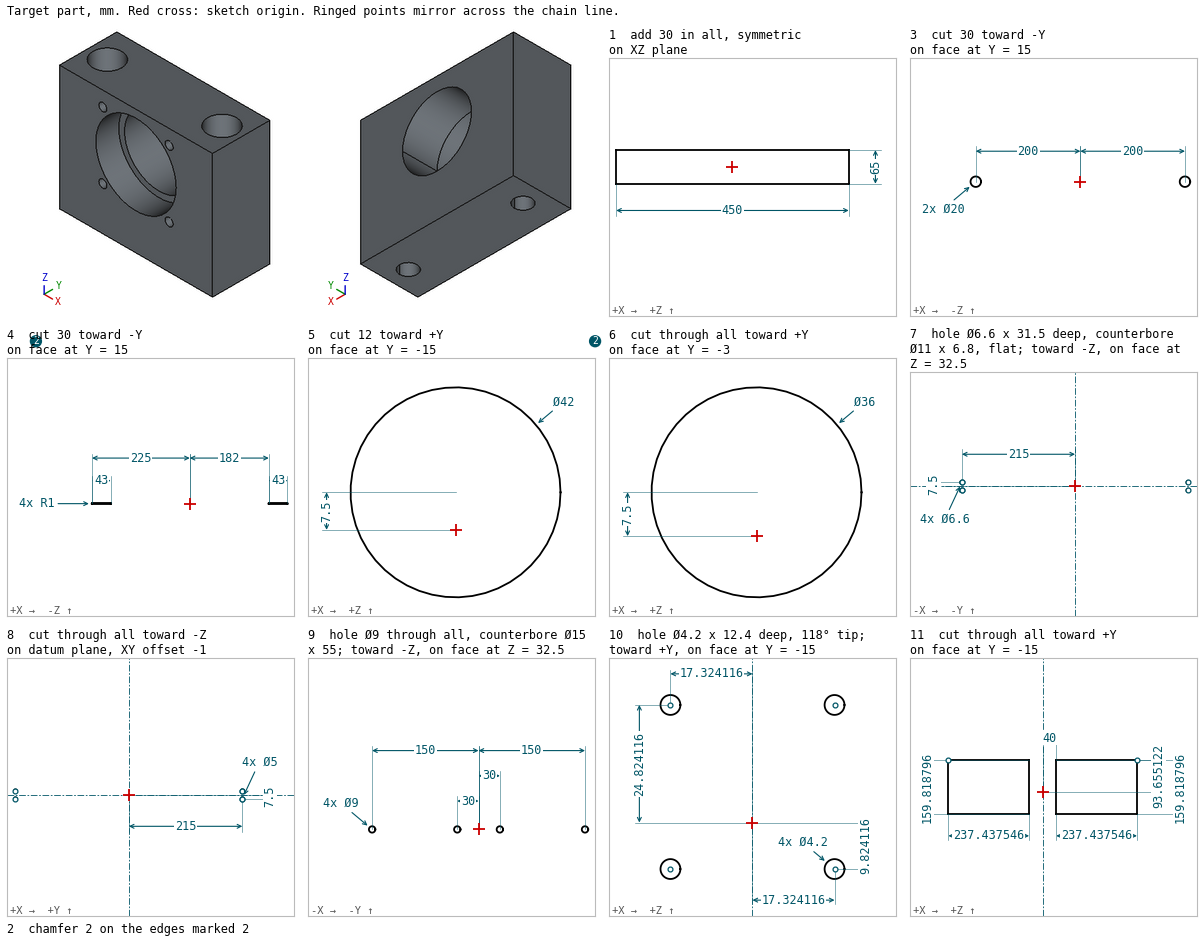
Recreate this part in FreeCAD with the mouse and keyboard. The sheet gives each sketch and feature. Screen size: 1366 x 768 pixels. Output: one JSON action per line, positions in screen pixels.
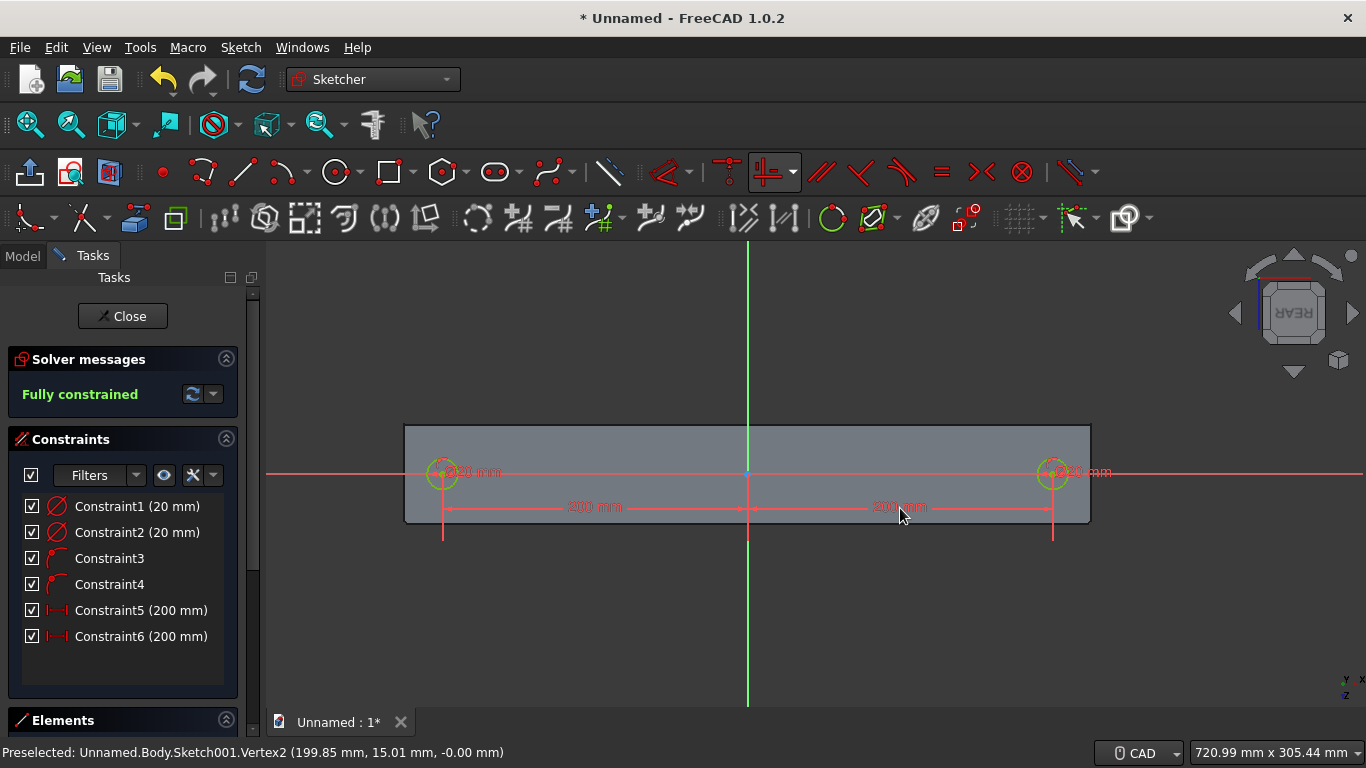
{"action": "left_click", "coordinate": [123, 316]}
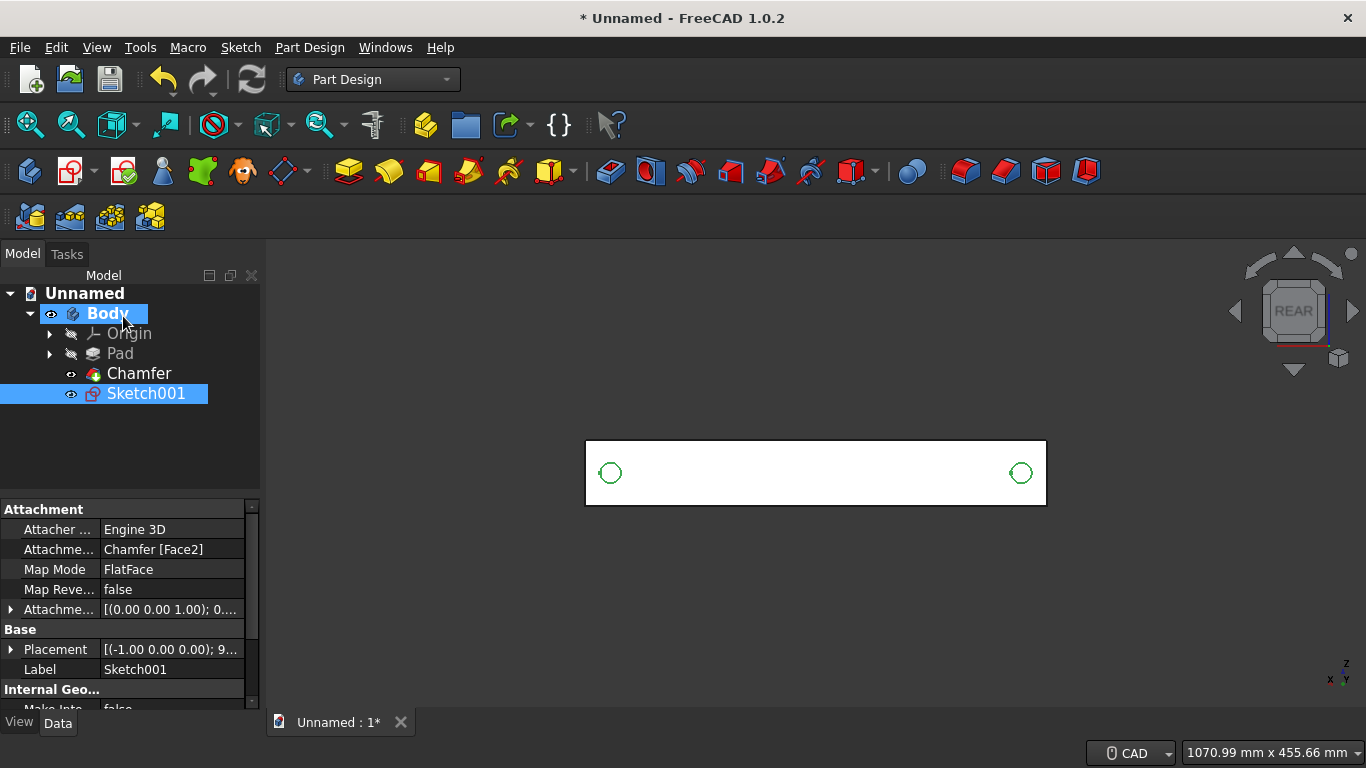
{"action": "left_click", "coordinate": [612, 172]}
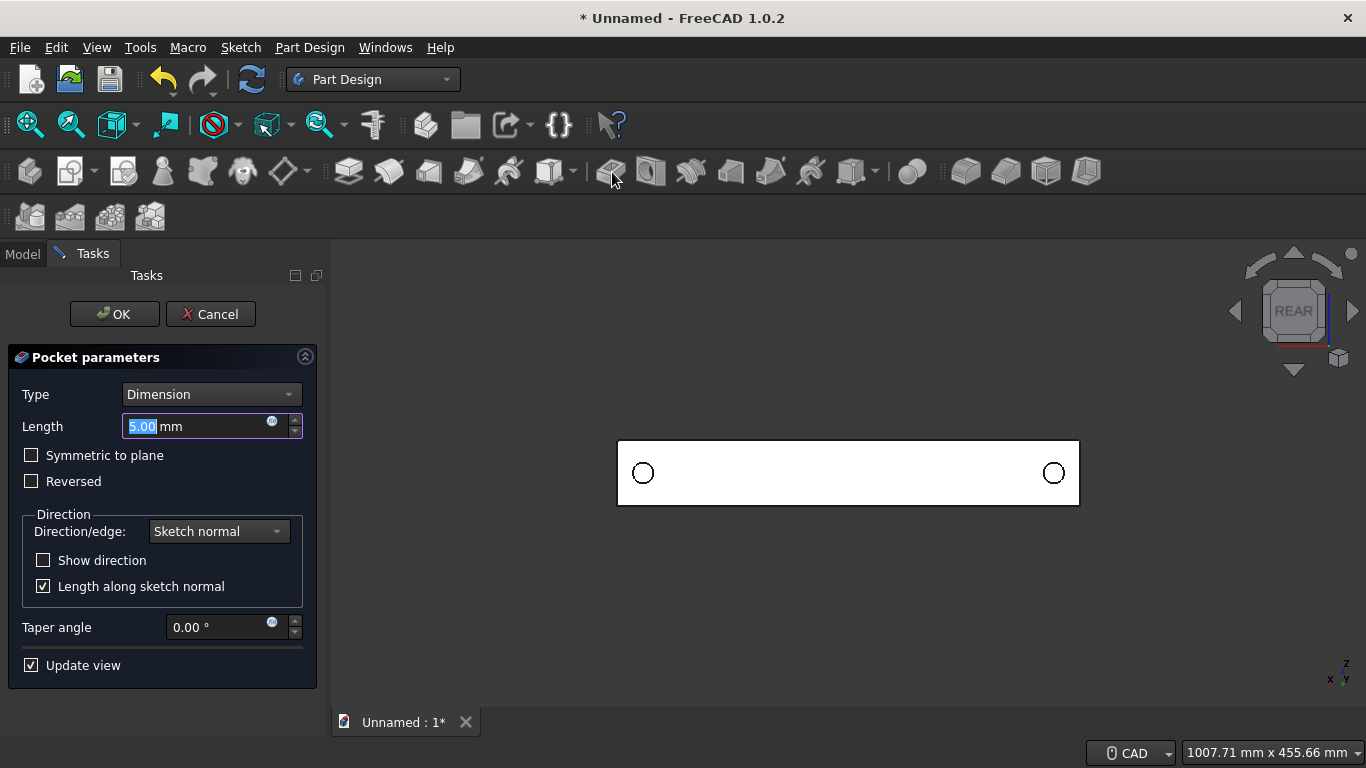
{"action": "type", "text": "30"}
{"action": "key", "text": "Tab"}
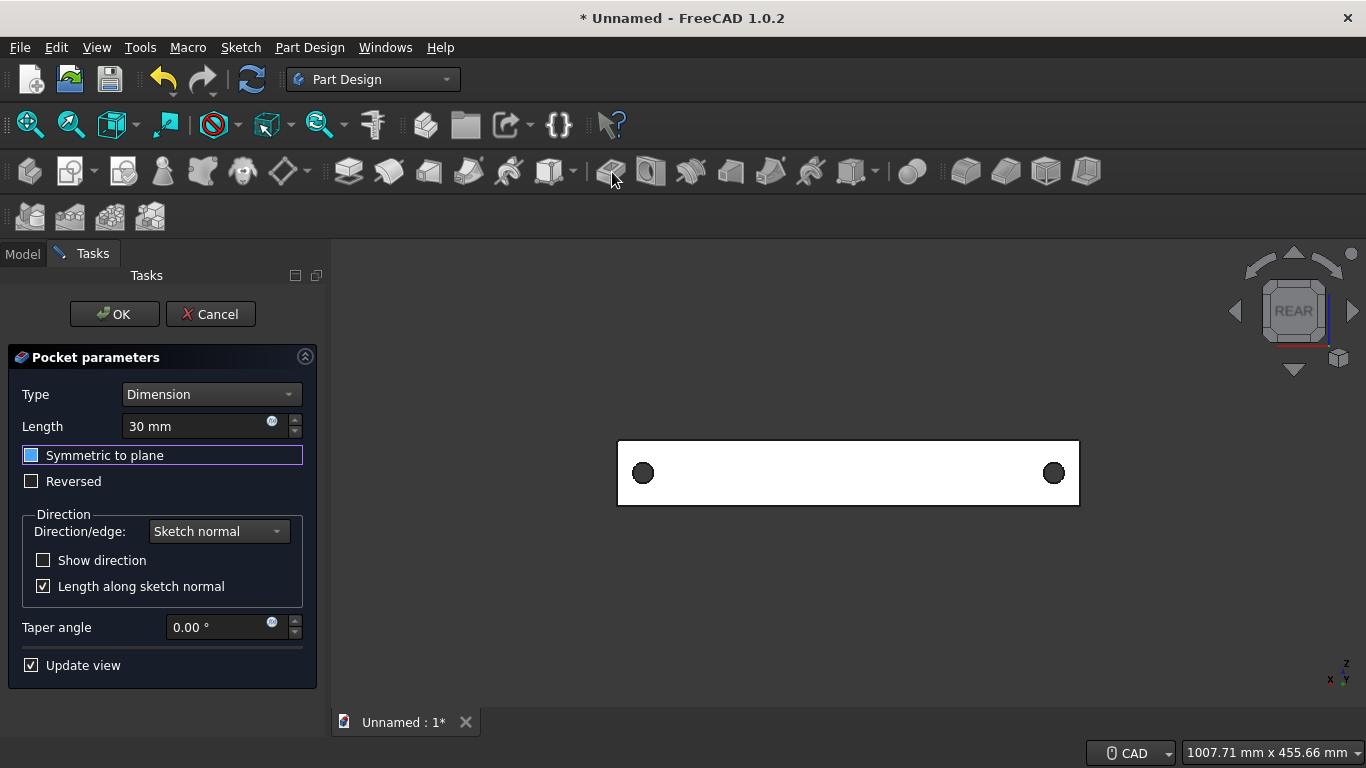
{"action": "left_click", "coordinate": [115, 314]}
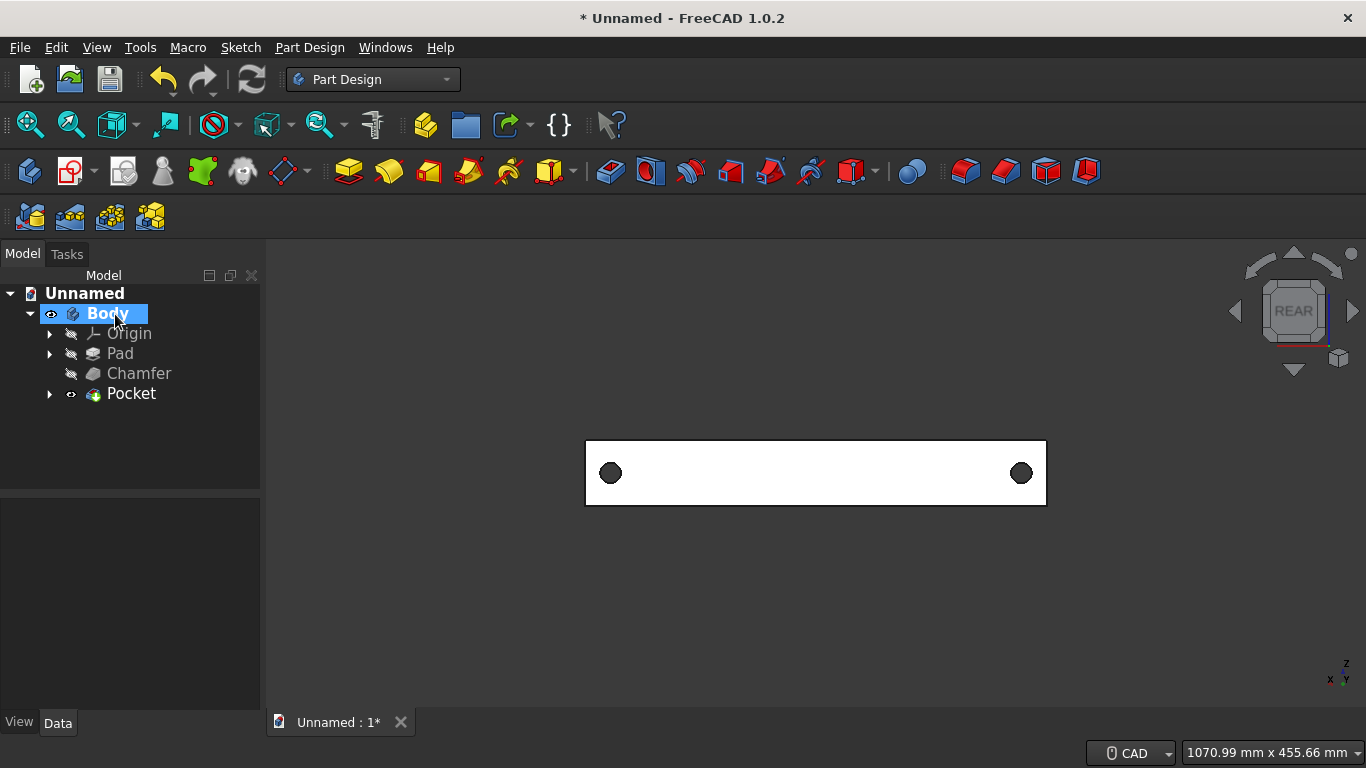
{"action": "key", "text": "v f"}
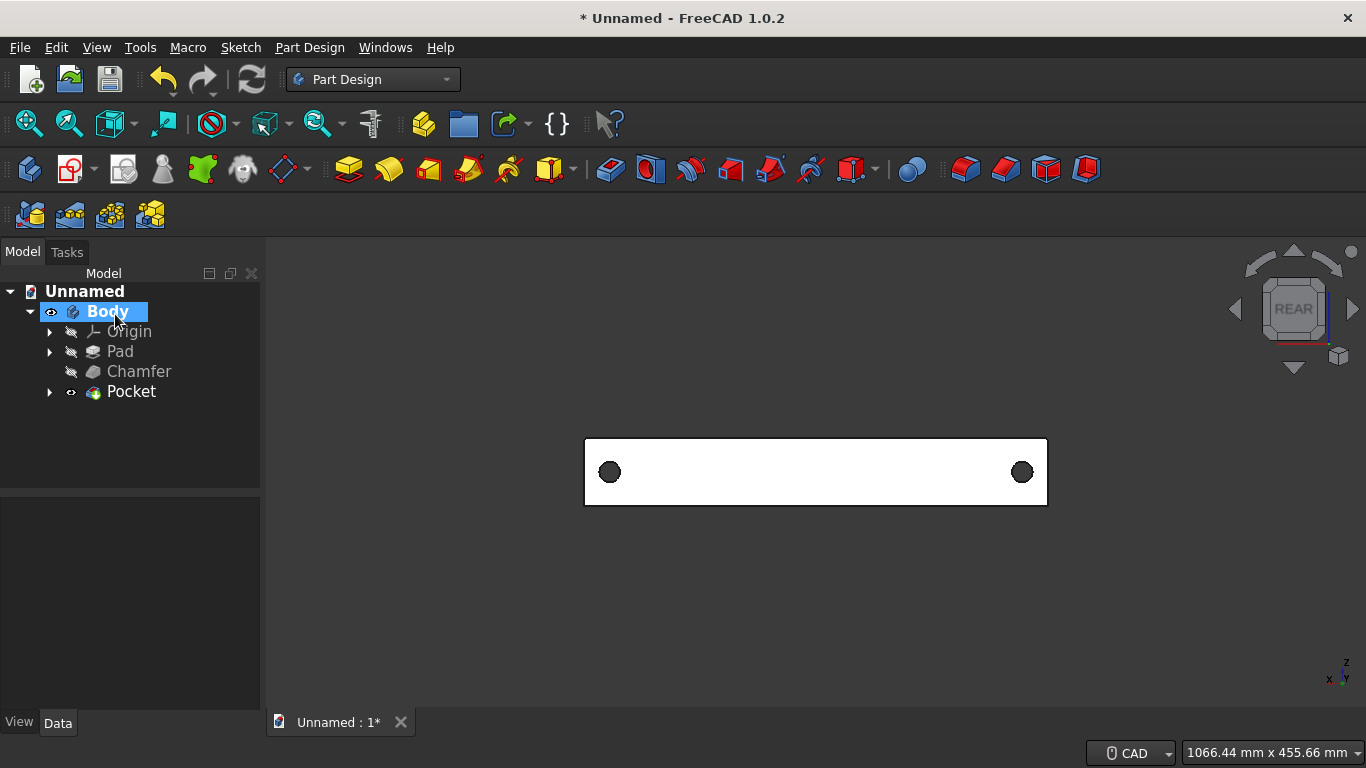
{"action": "left_click", "coordinate": [683, 471]}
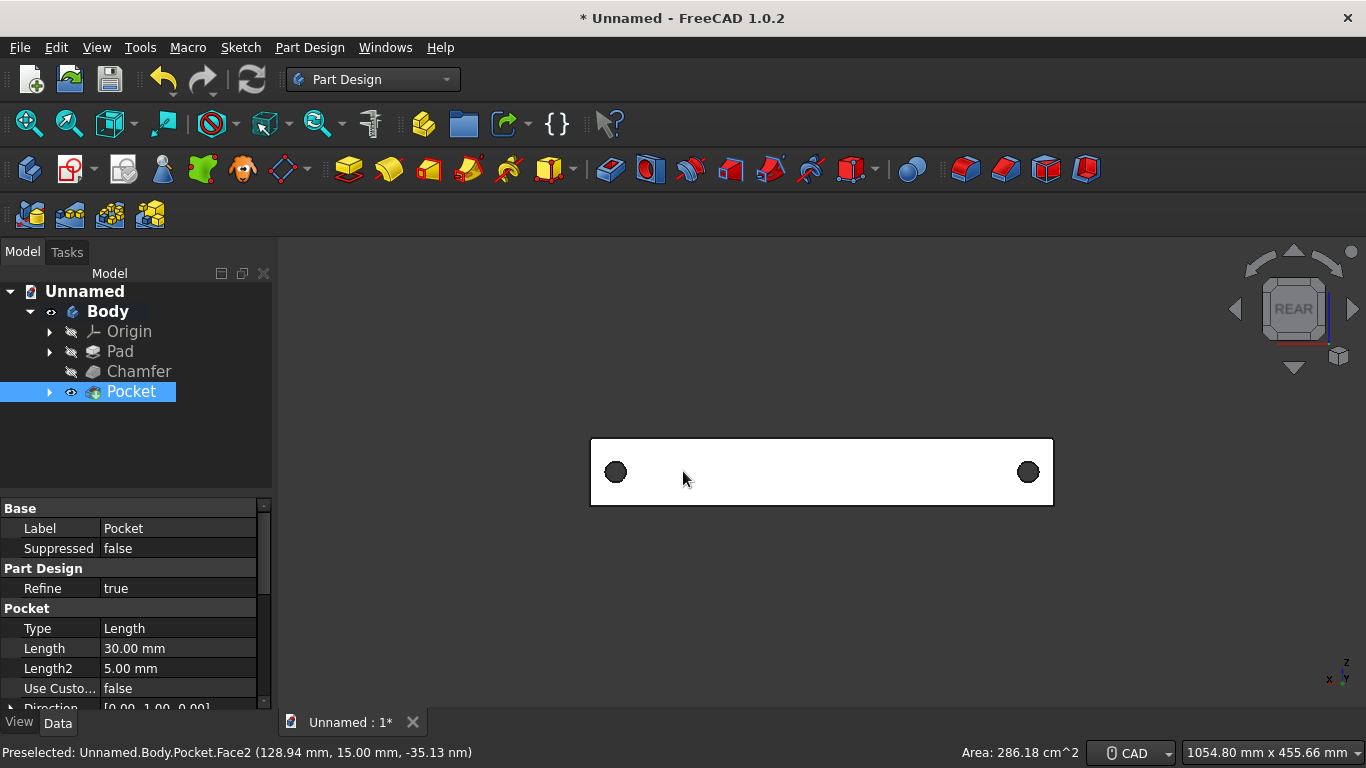
{"action": "left_click", "coordinate": [70, 170]}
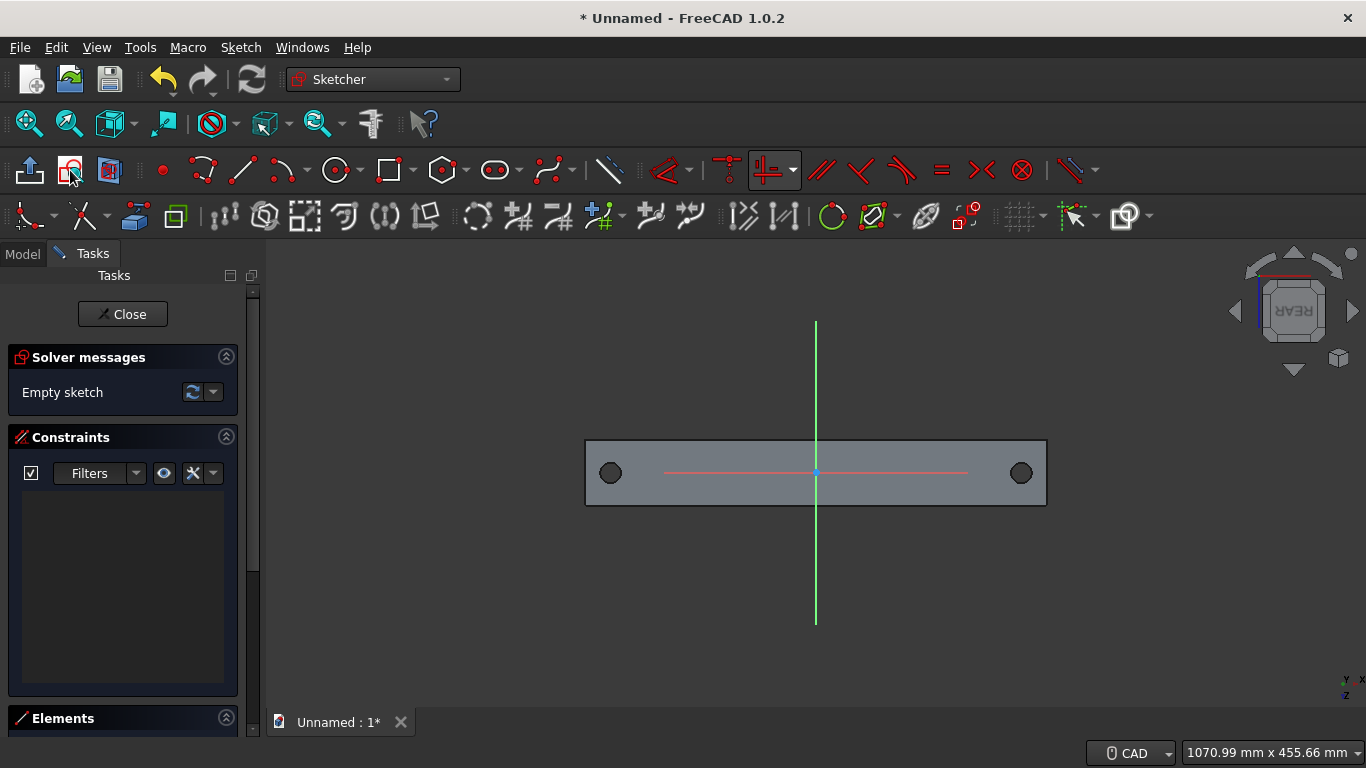
{"action": "scroll", "coordinate": [955, 473], "scroll_direction": "up", "scroll_amount": 2}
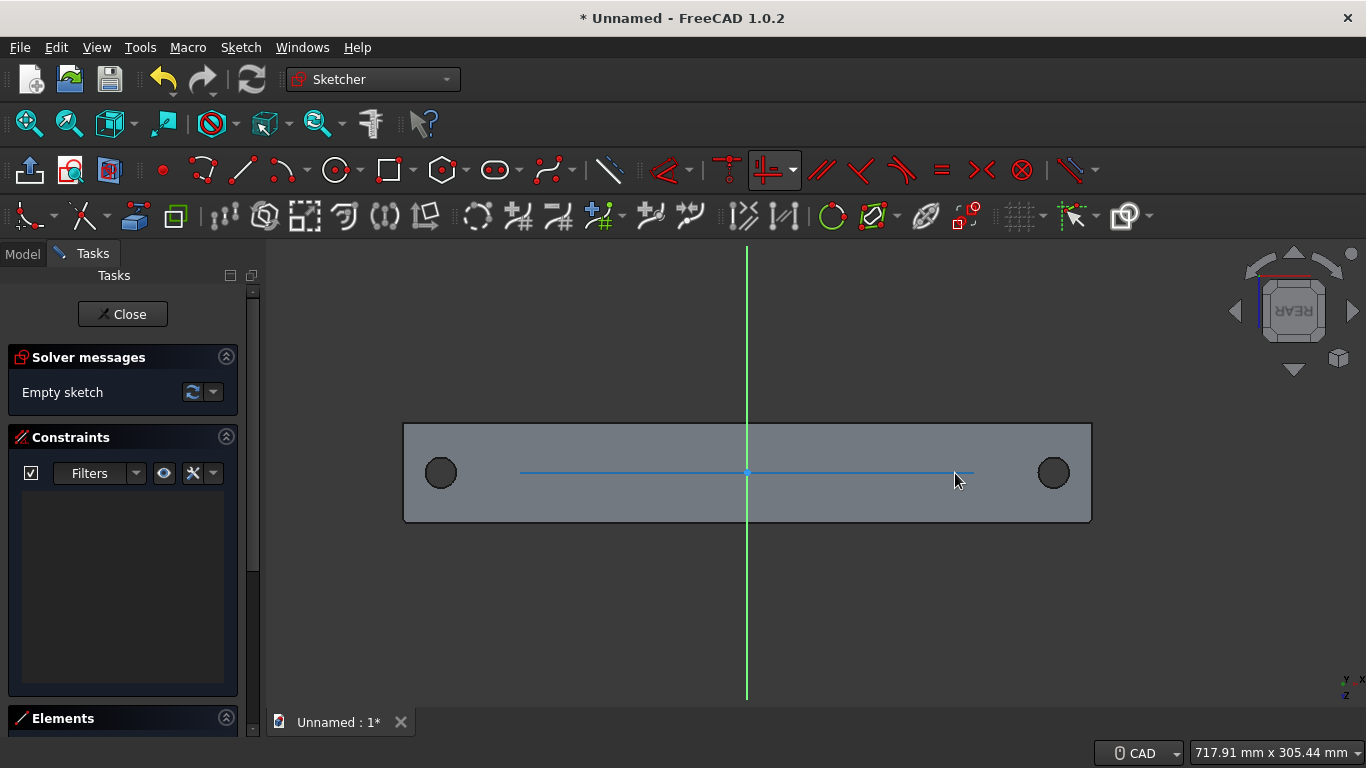
{"action": "key", "text": "g s"}